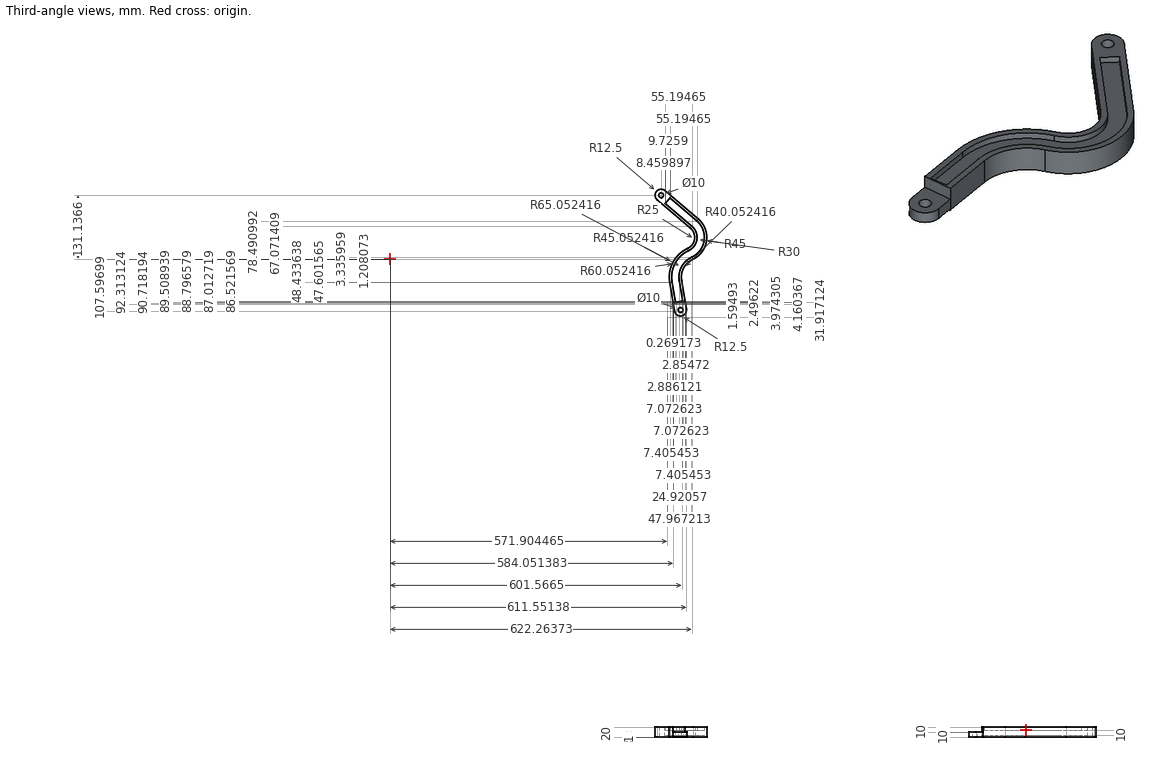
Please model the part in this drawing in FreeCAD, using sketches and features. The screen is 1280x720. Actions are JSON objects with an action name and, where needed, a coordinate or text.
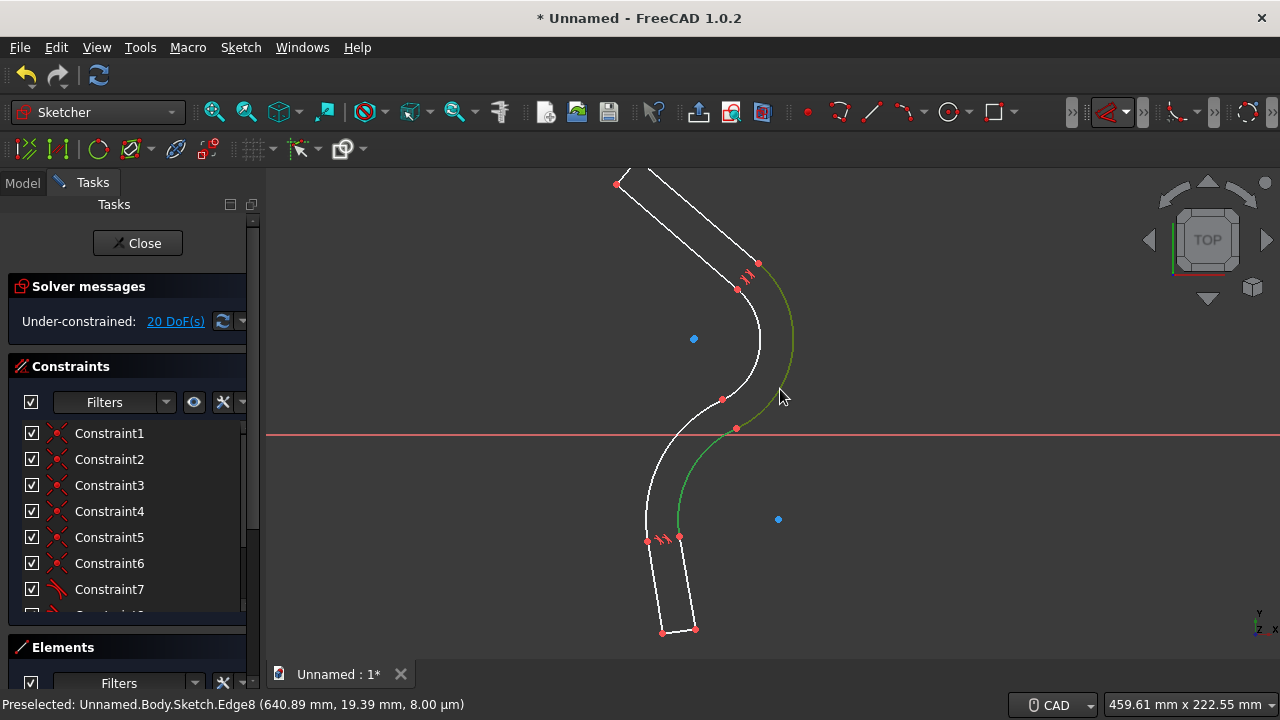
{"action": "key", "text": "t"}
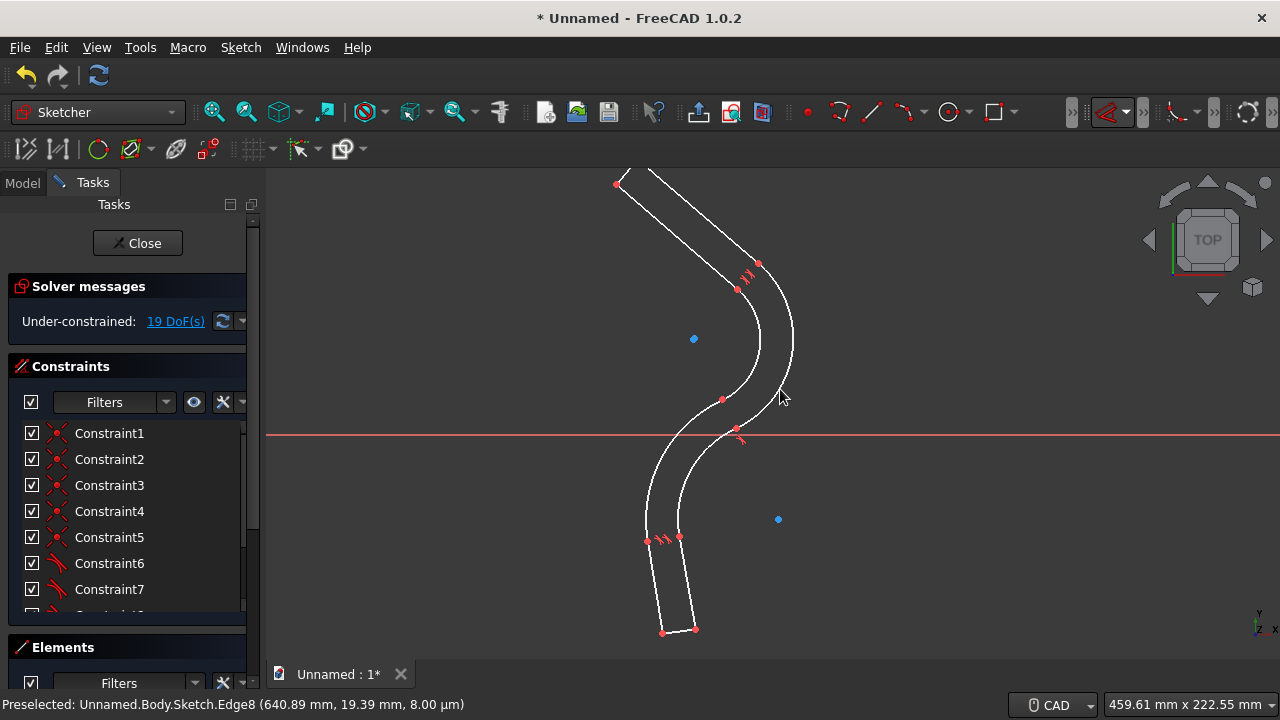
{"action": "left_click", "coordinate": [751, 373]}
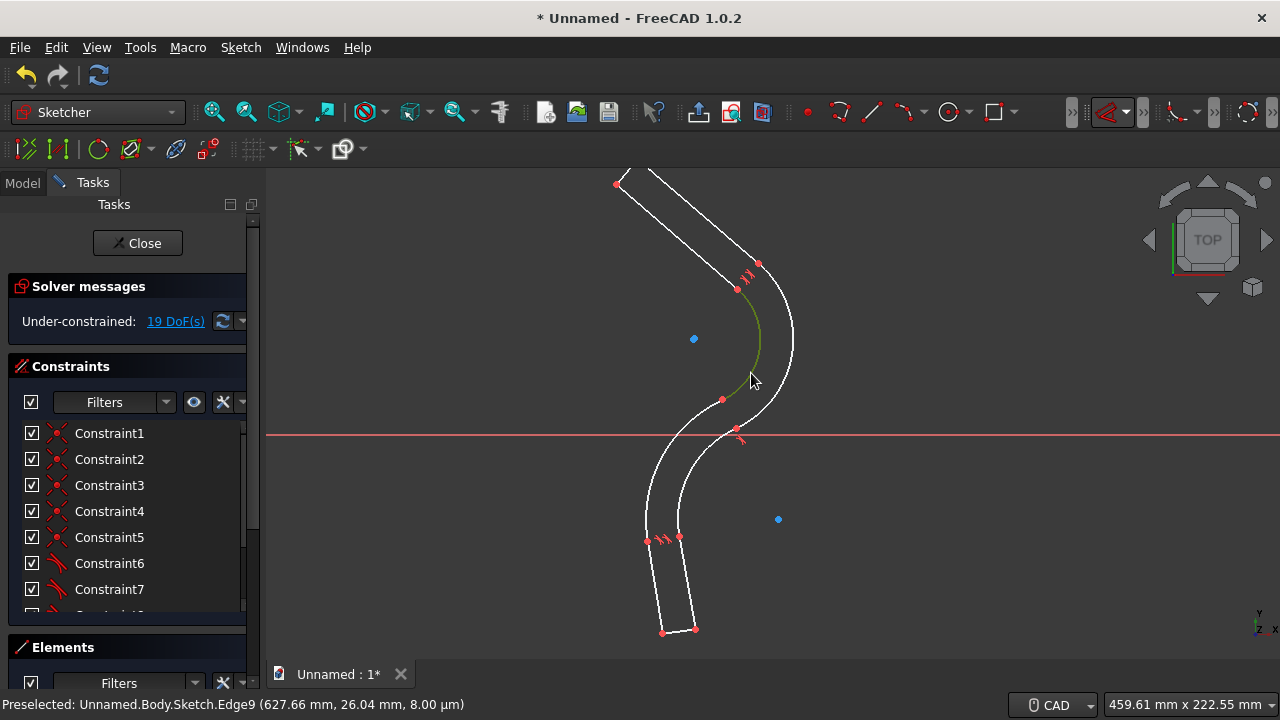
{"action": "left_click", "coordinate": [650, 490]}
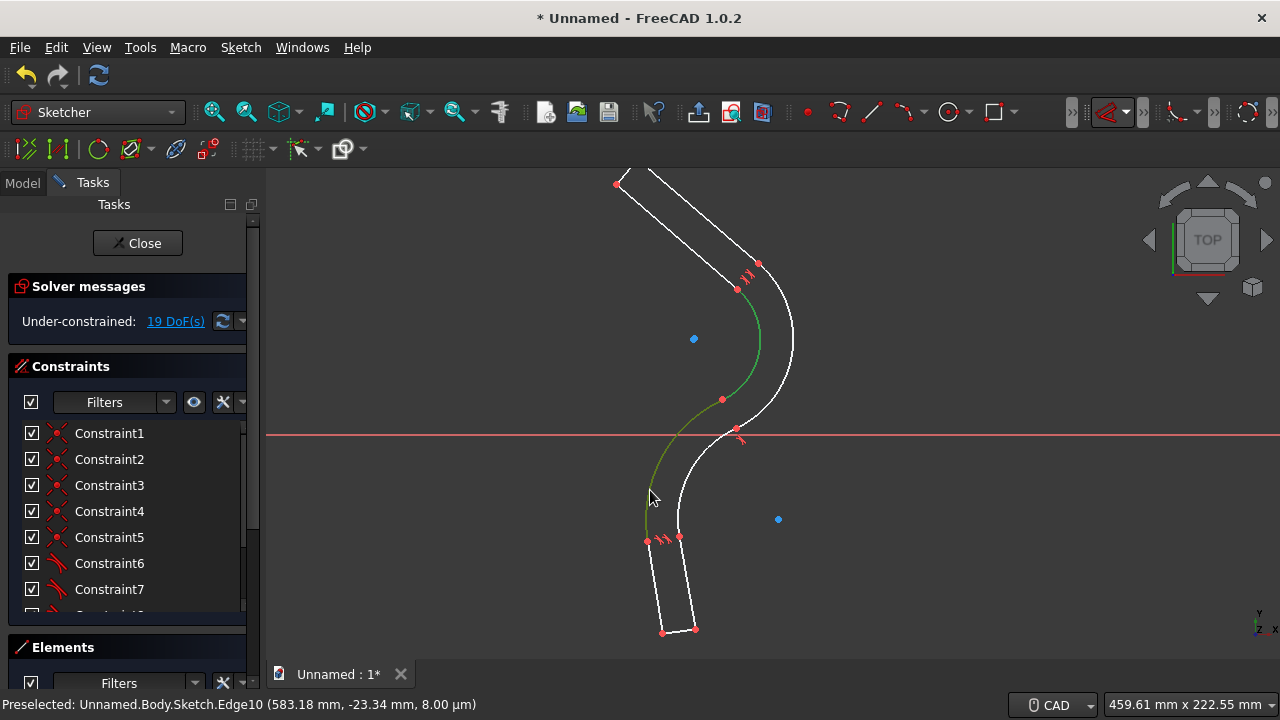
{"action": "key", "text": "t"}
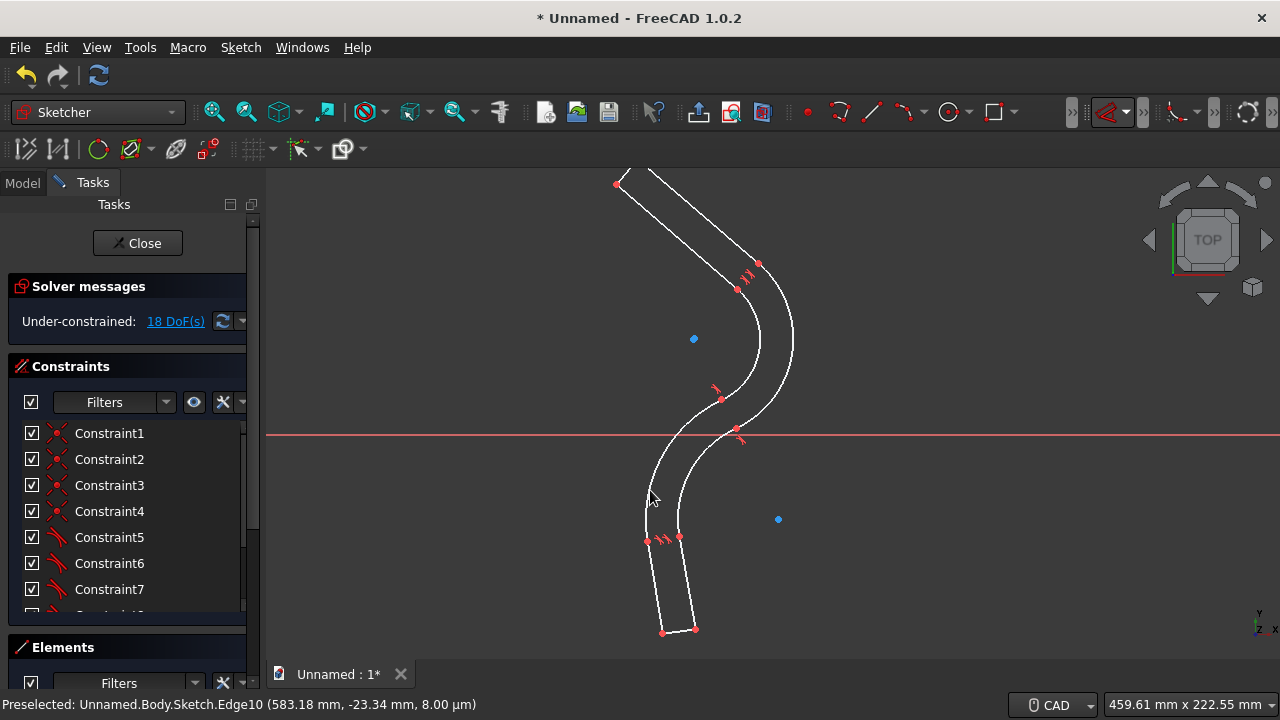
{"action": "left_click", "coordinate": [779, 389]}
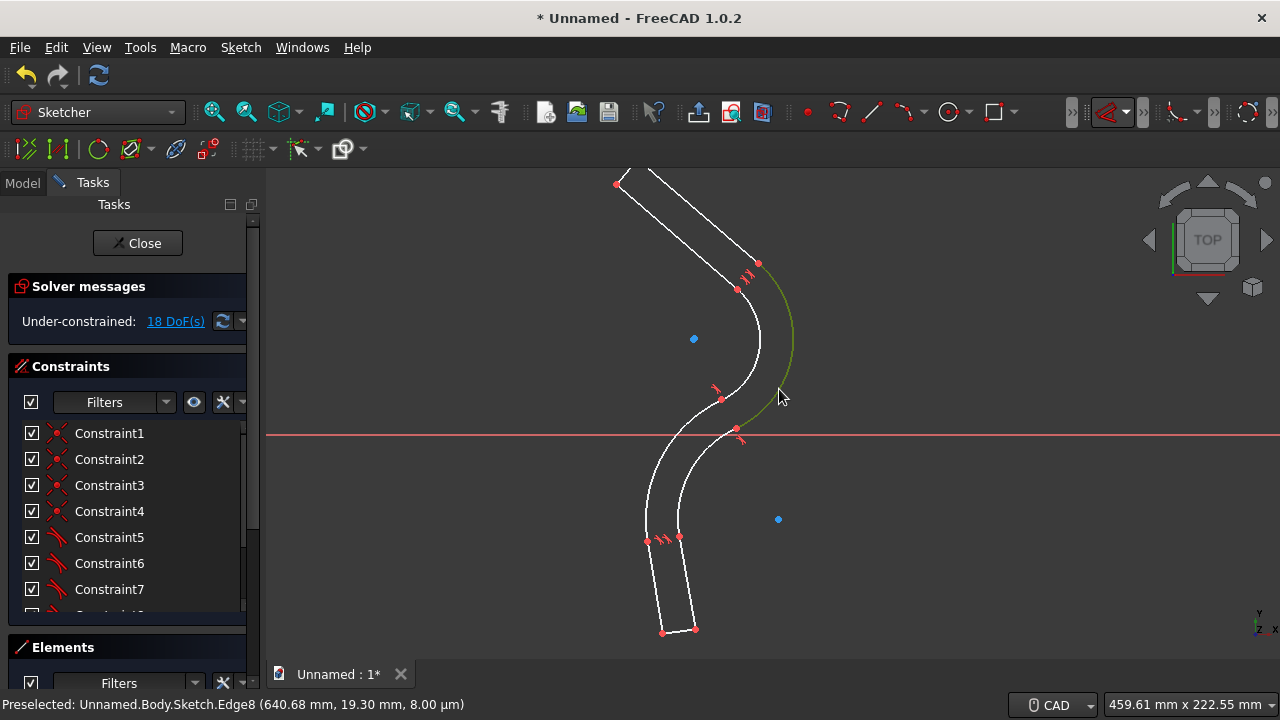
{"action": "left_click", "coordinate": [751, 374]}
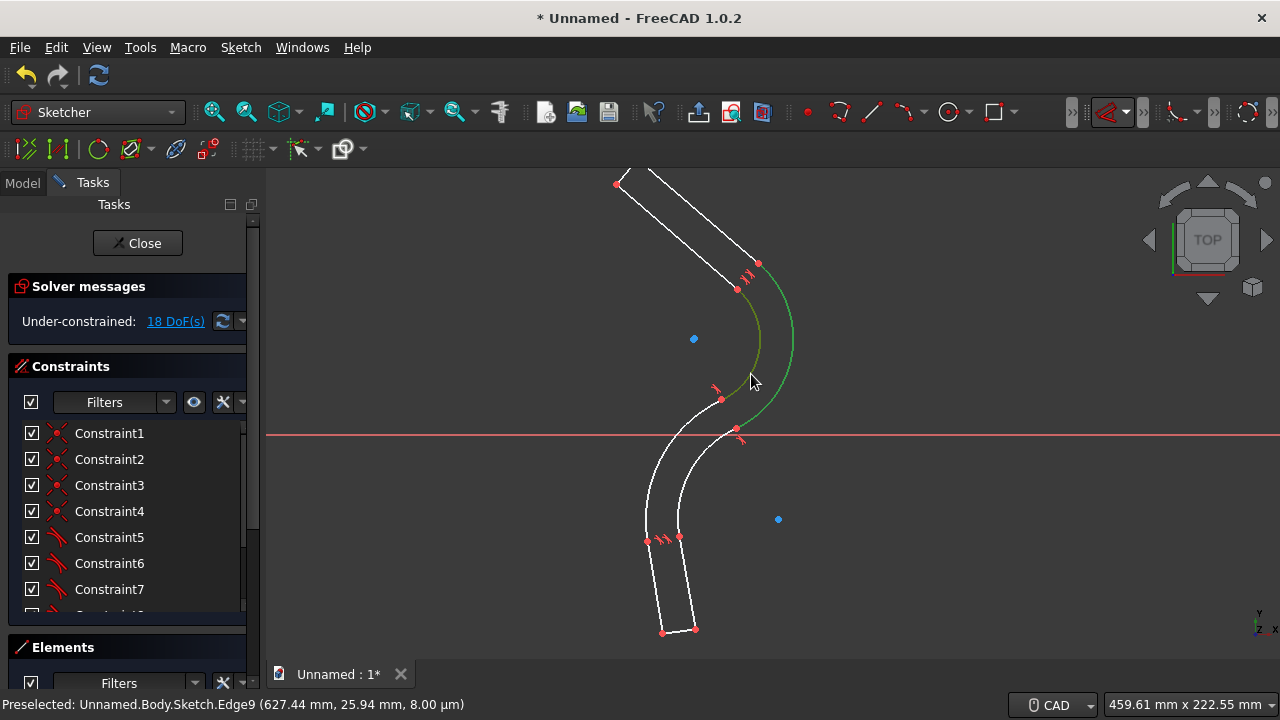
{"action": "key", "text": "c"}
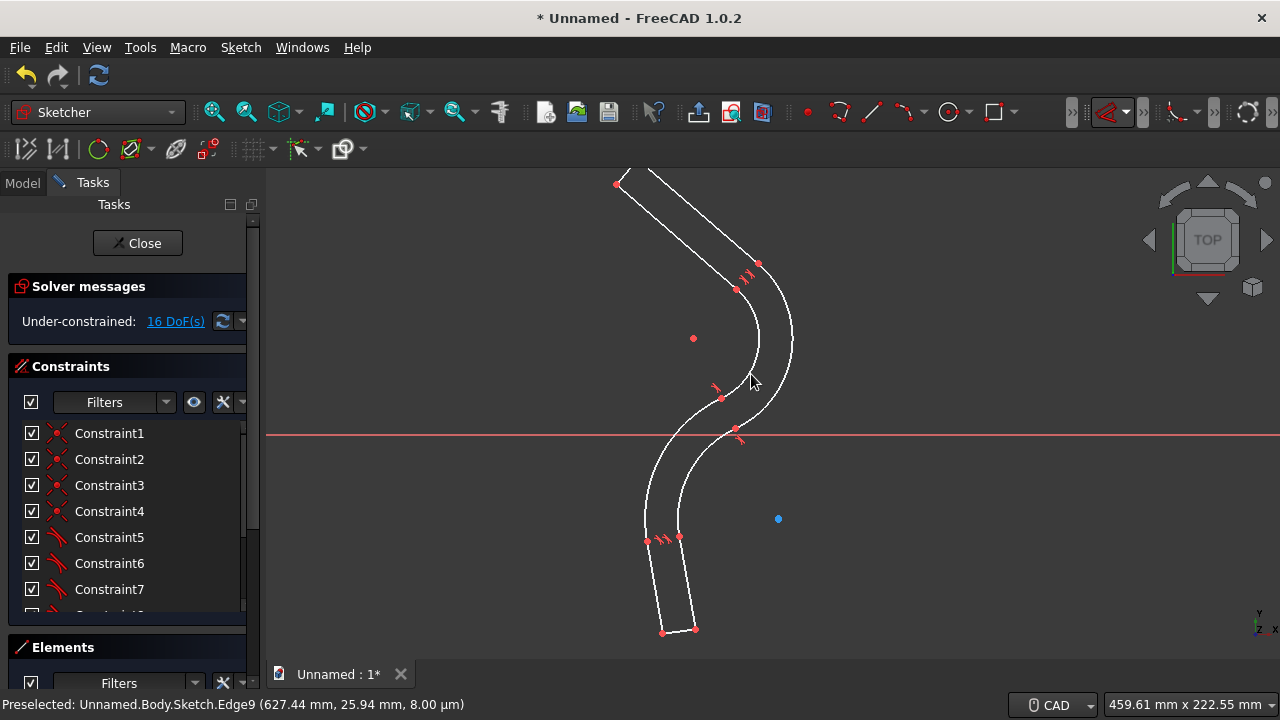
{"action": "left_click", "coordinate": [704, 452]}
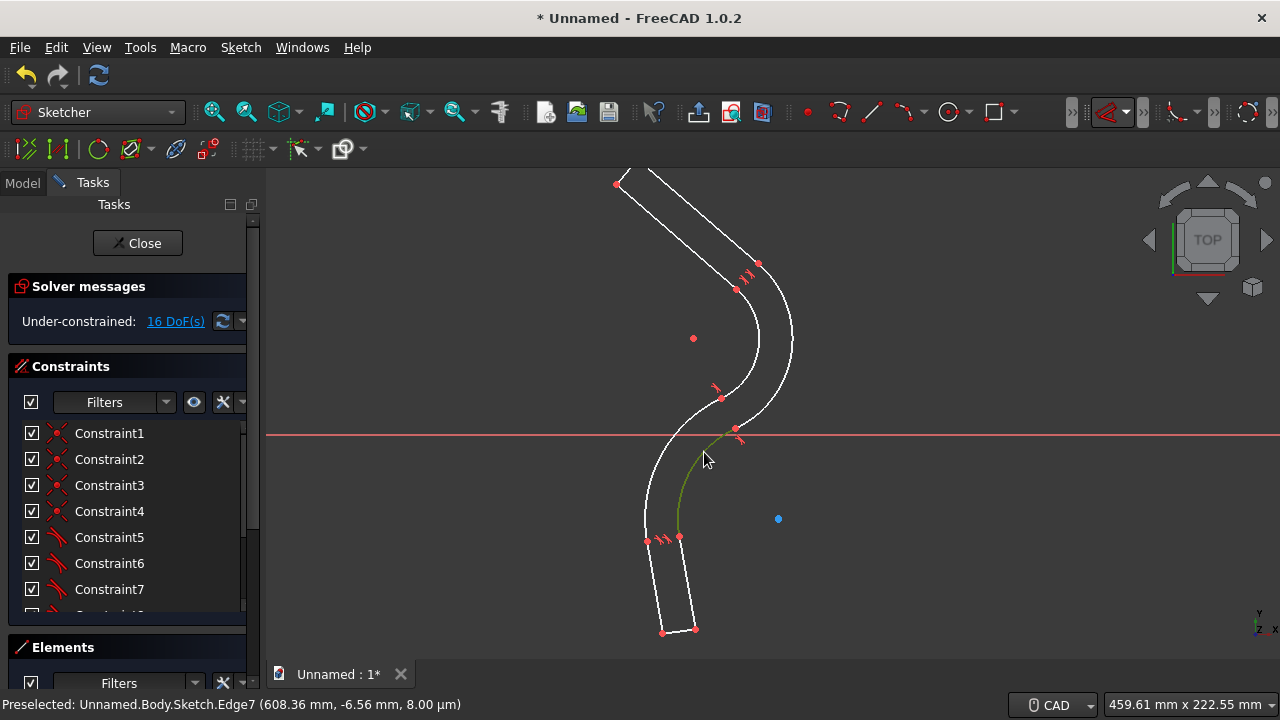
{"action": "left_click", "coordinate": [648, 490]}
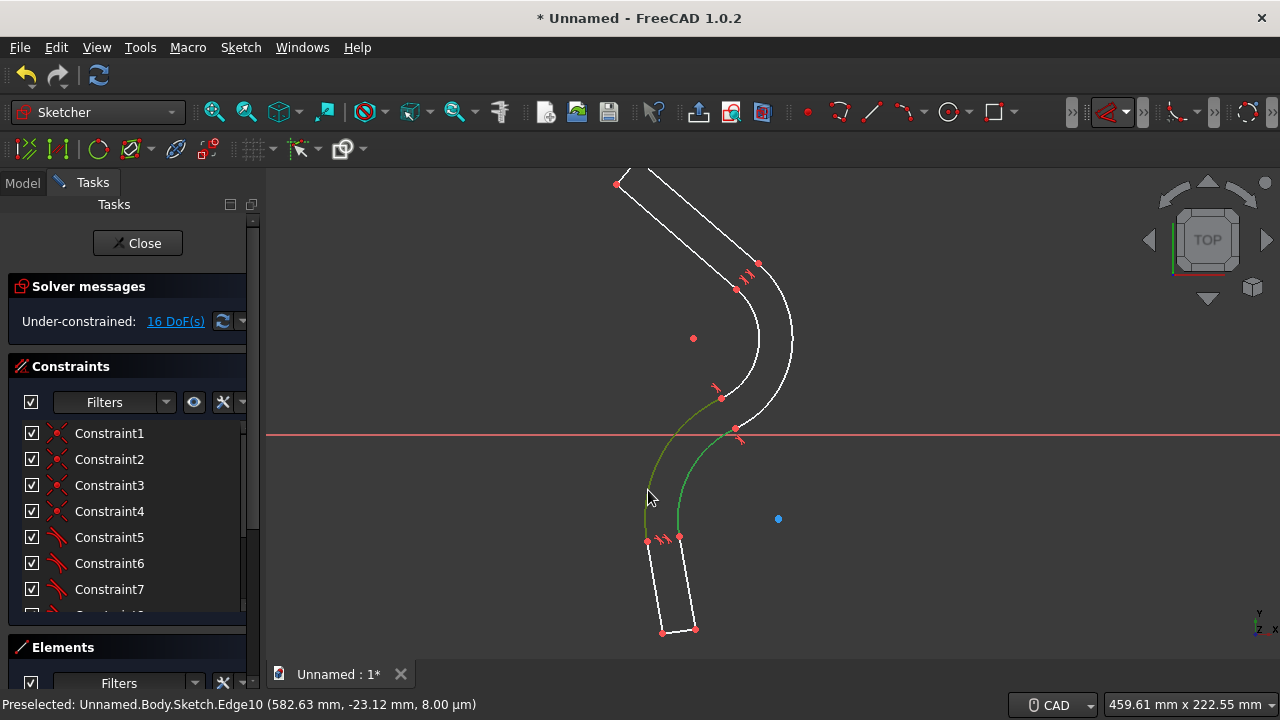
{"action": "key", "text": "c"}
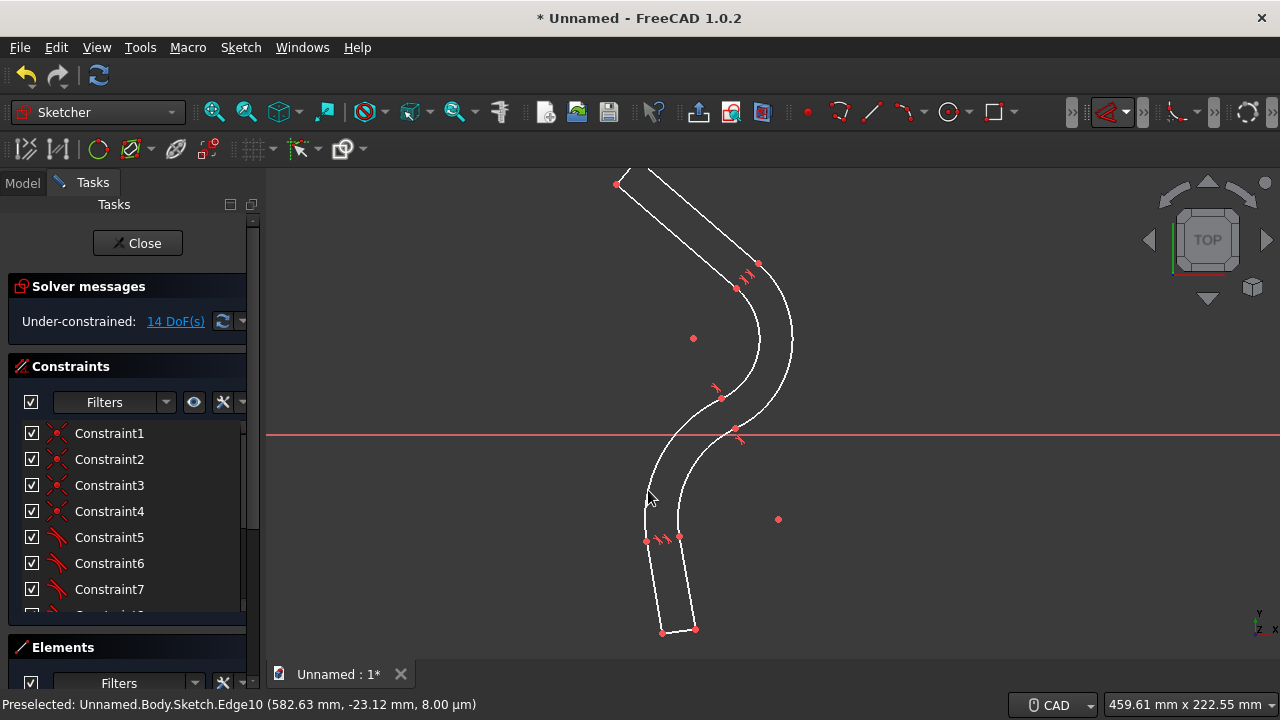
{"action": "left_click", "coordinate": [704, 452]}